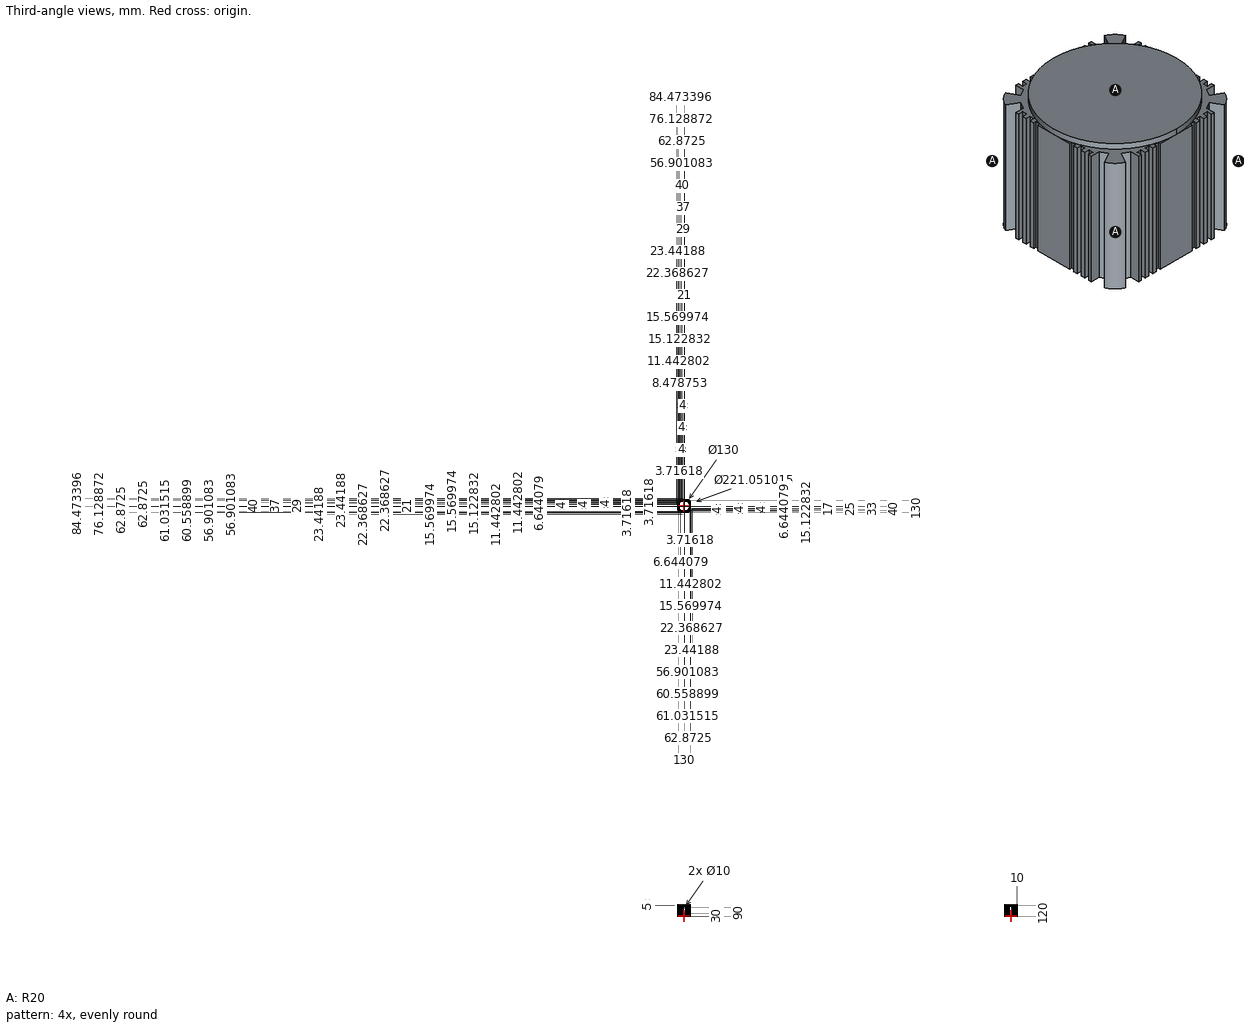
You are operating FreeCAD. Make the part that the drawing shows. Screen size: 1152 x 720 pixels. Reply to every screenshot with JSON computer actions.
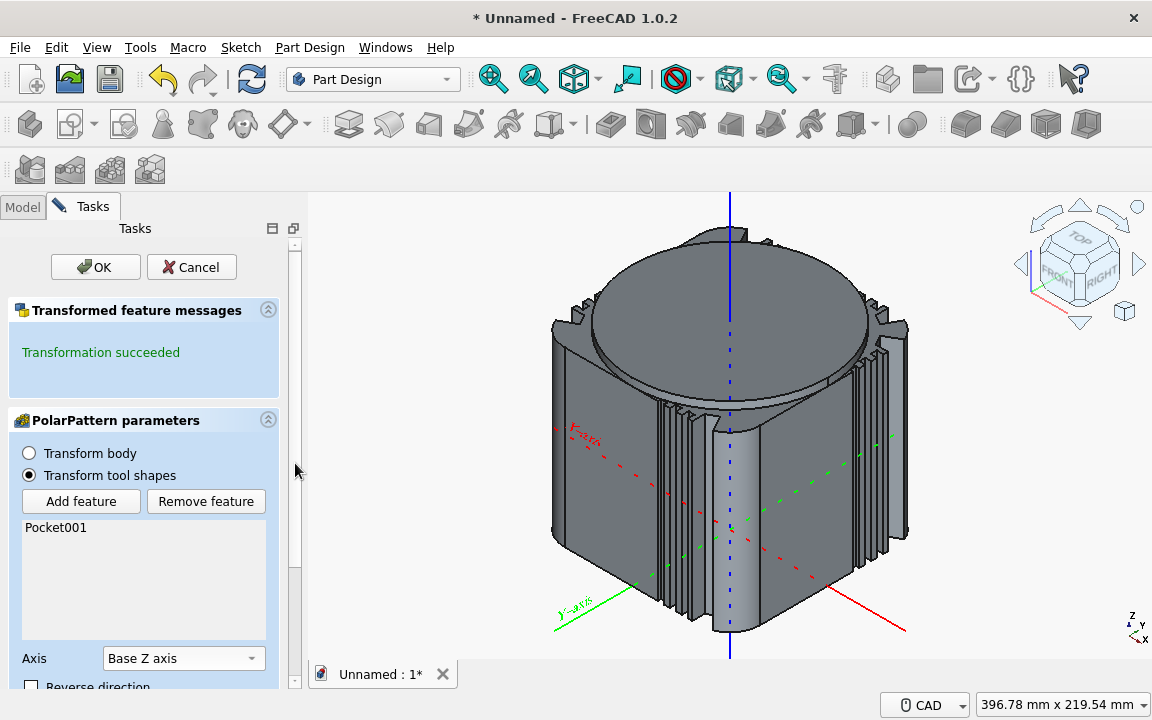
{"action": "left_click", "coordinate": [96, 267]}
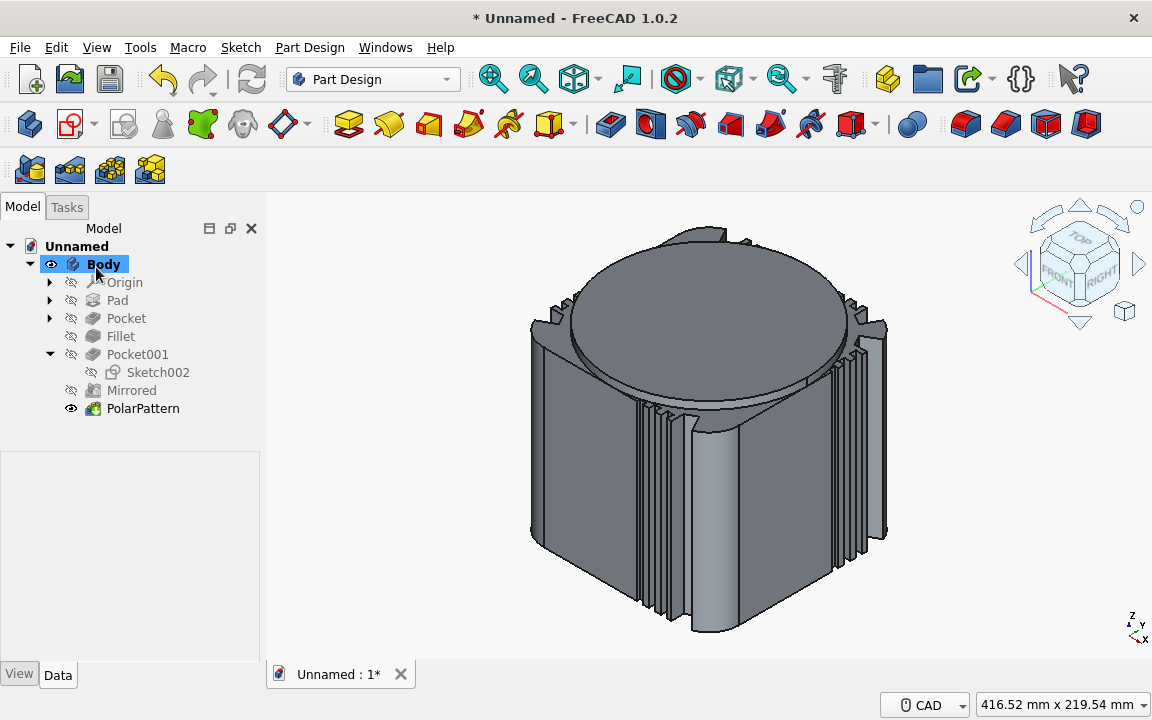
{"action": "left_click", "coordinate": [709, 418]}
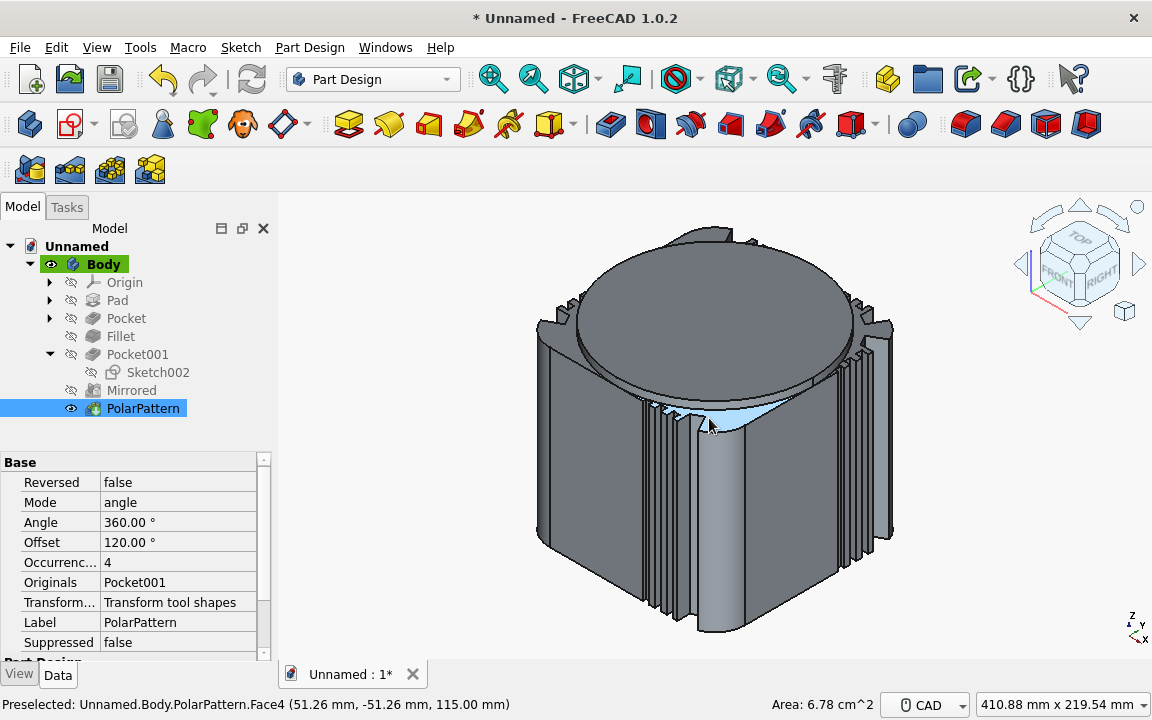
{"action": "left_click", "coordinate": [70, 124]}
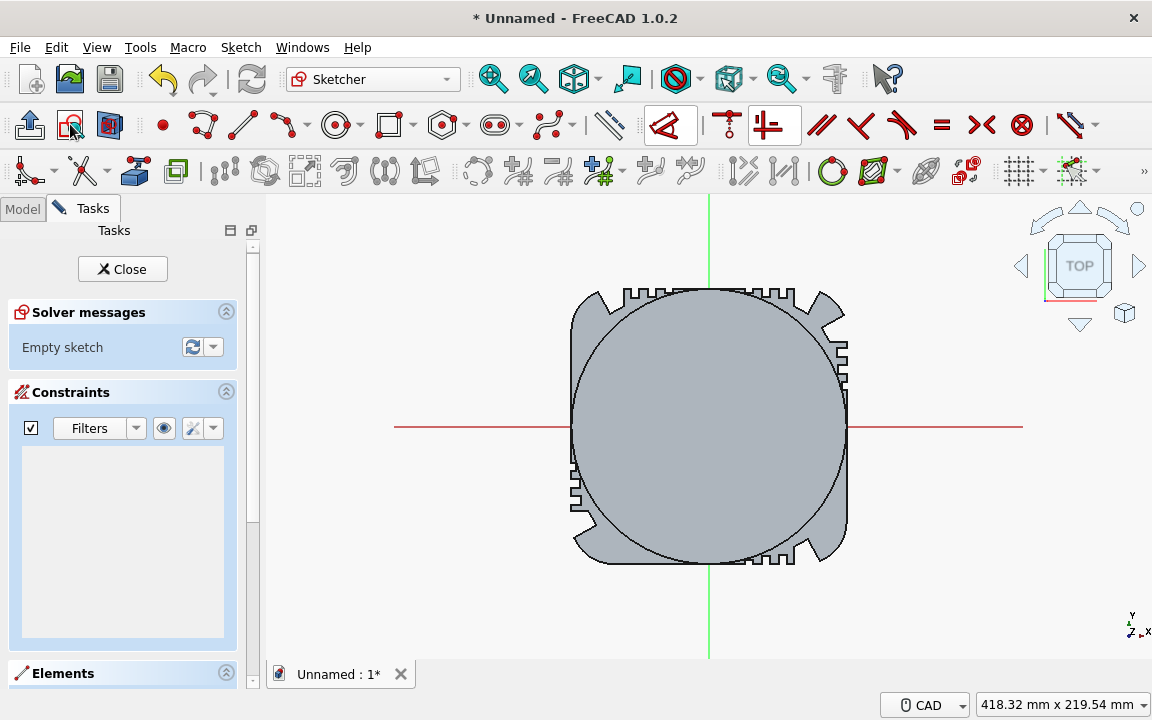
{"action": "scroll", "coordinate": [606, 334], "scroll_direction": "up", "scroll_amount": 5}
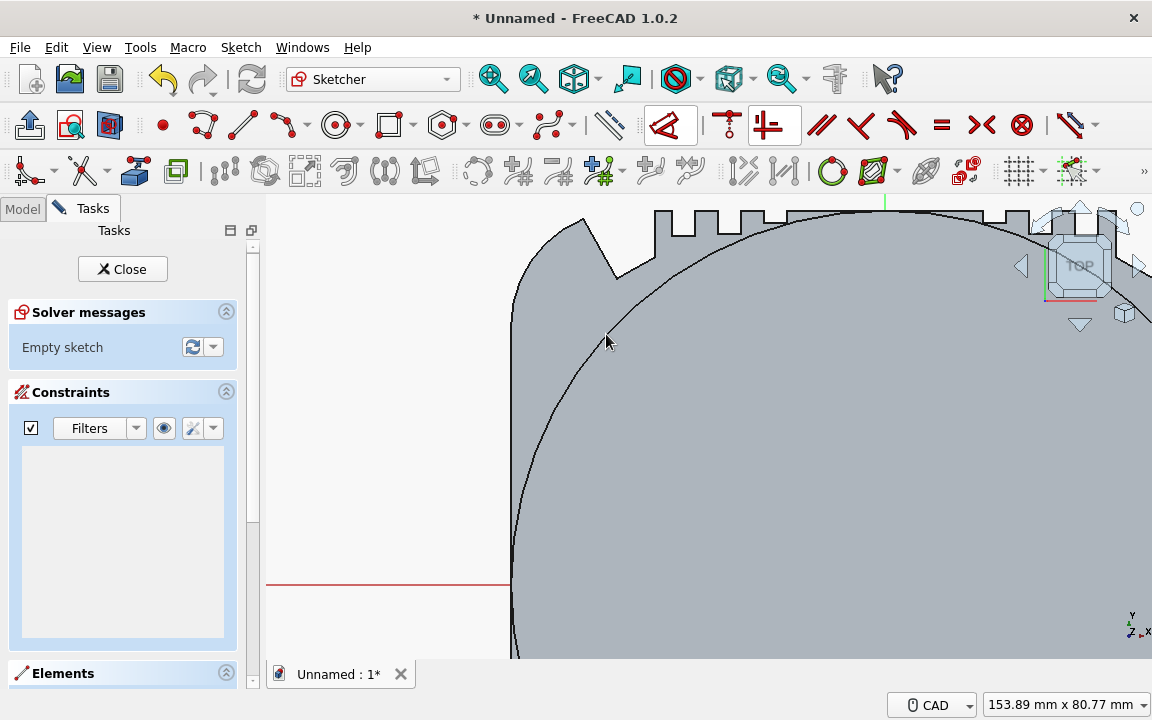
{"action": "left_click", "coordinate": [204, 126]}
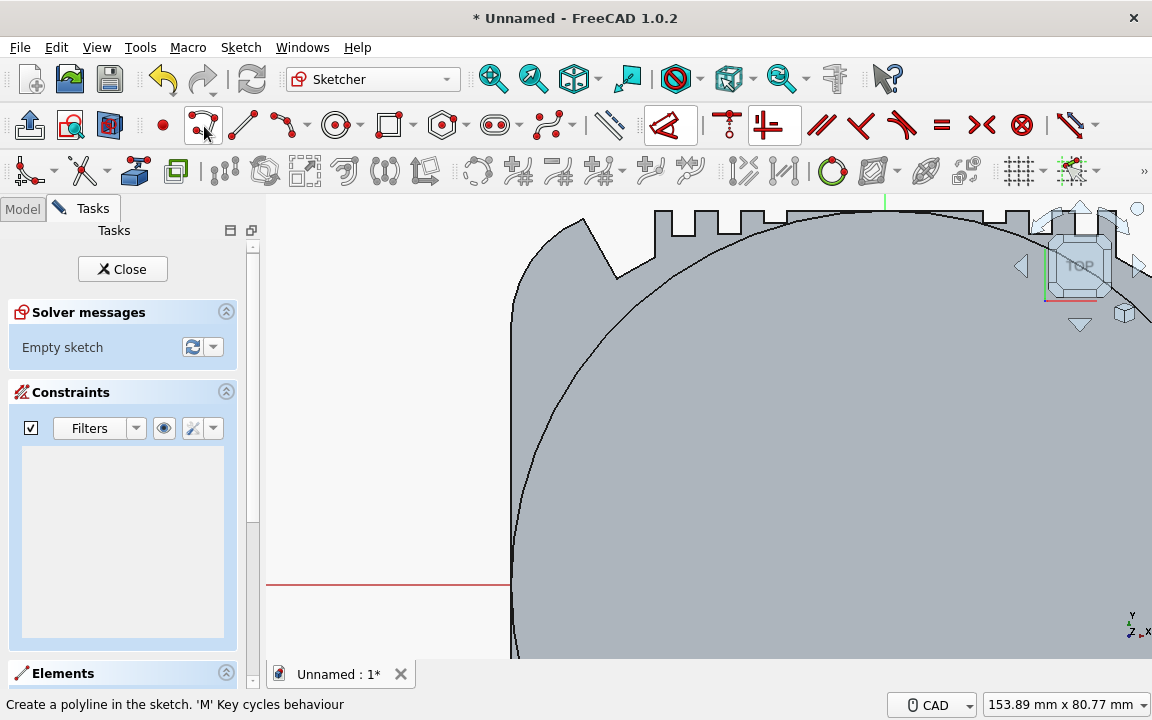
{"action": "left_click", "coordinate": [558, 355]}
{"action": "left_click", "coordinate": [579, 316]}
{"action": "left_click", "coordinate": [492, 268]}
{"action": "left_click", "coordinate": [492, 355]}
{"action": "left_click", "coordinate": [558, 356]}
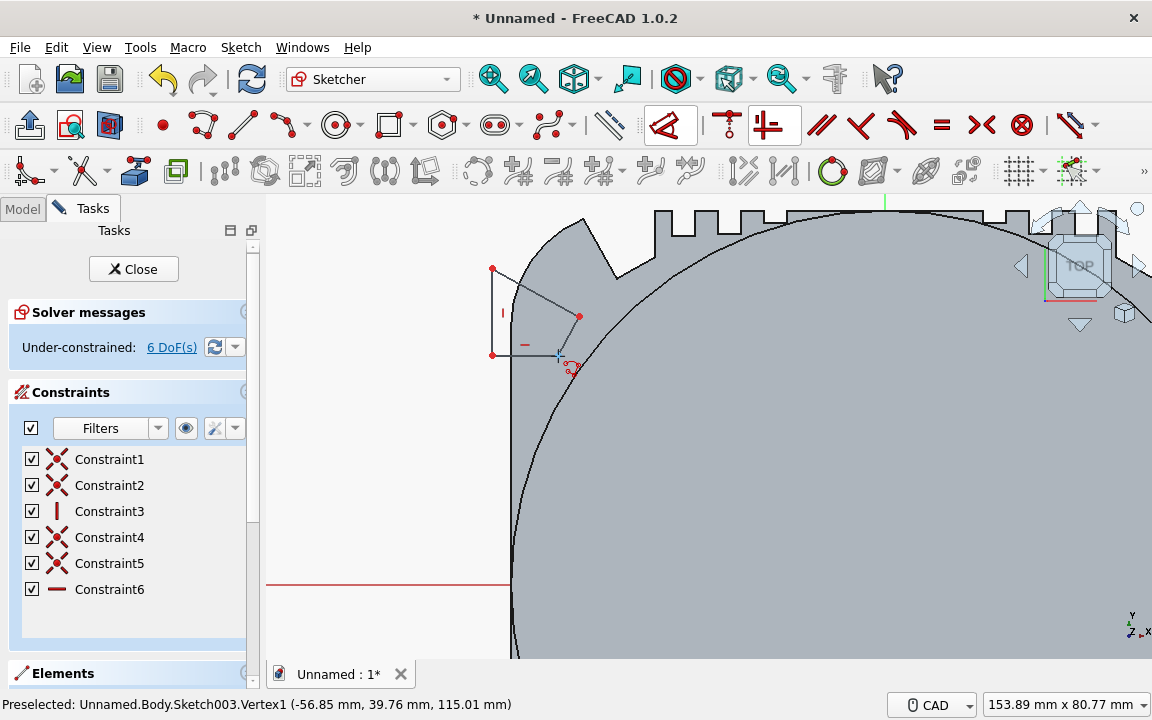
{"action": "left_click", "coordinate": [390, 126]}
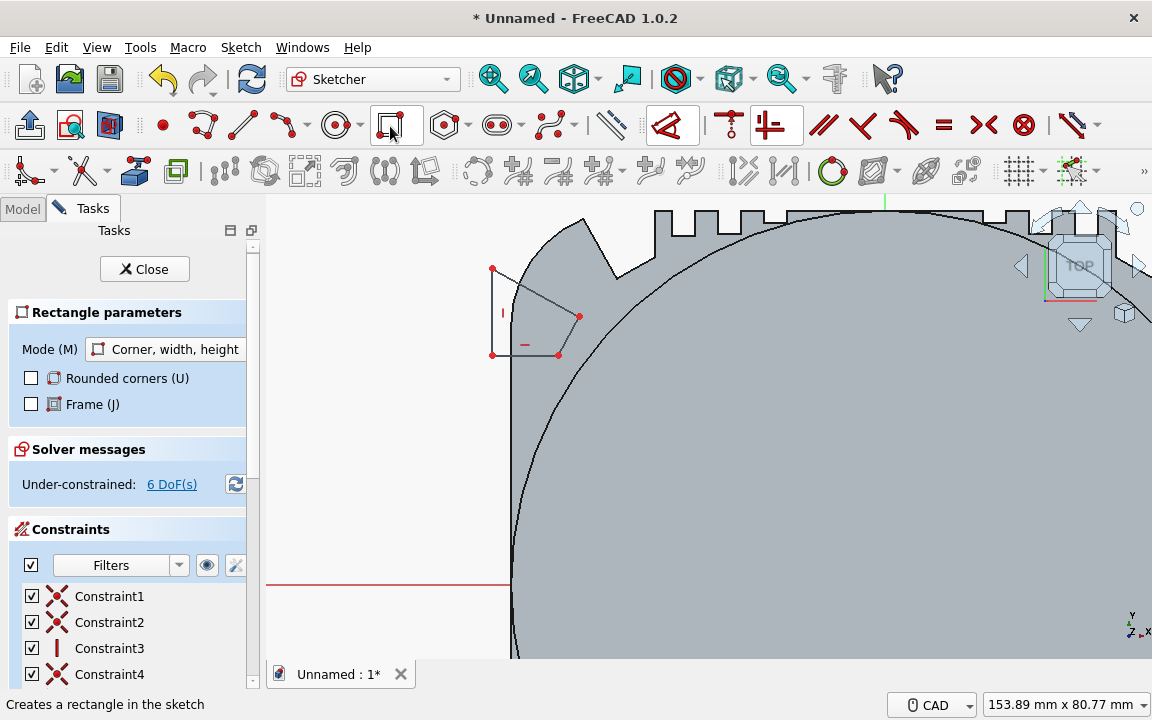
{"action": "left_click", "coordinate": [447, 372]}
{"action": "mouse_move", "coordinate": [537, 395]}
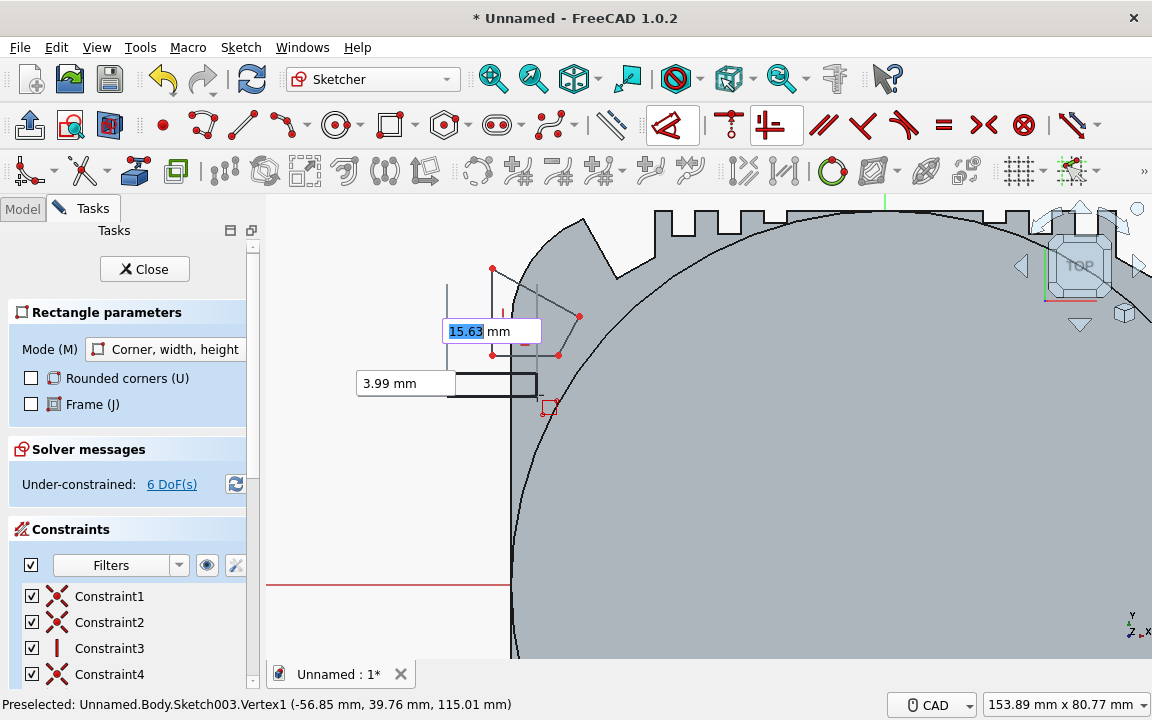
{"action": "type", "text": "15.569974"}
{"action": "key", "text": "Tab"}
{"action": "type", "text": "4"}
{"action": "key", "text": "Return"}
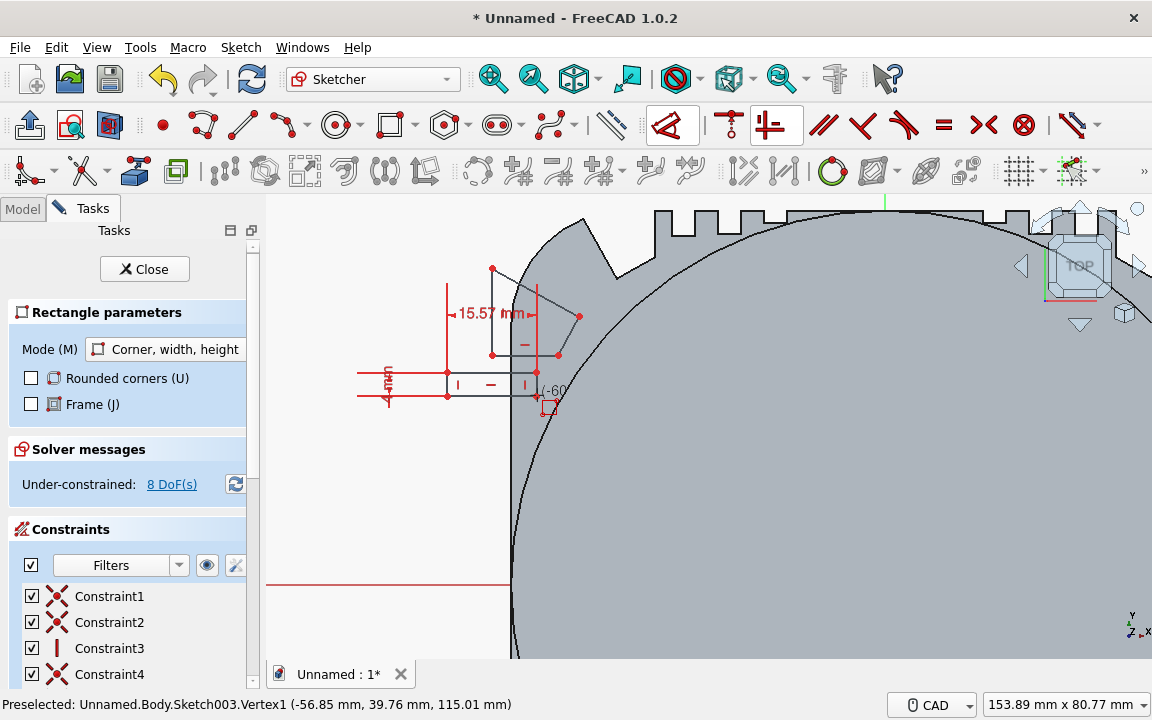
{"action": "left_click", "coordinate": [399, 418]}
{"action": "mouse_move", "coordinate": [534, 441]}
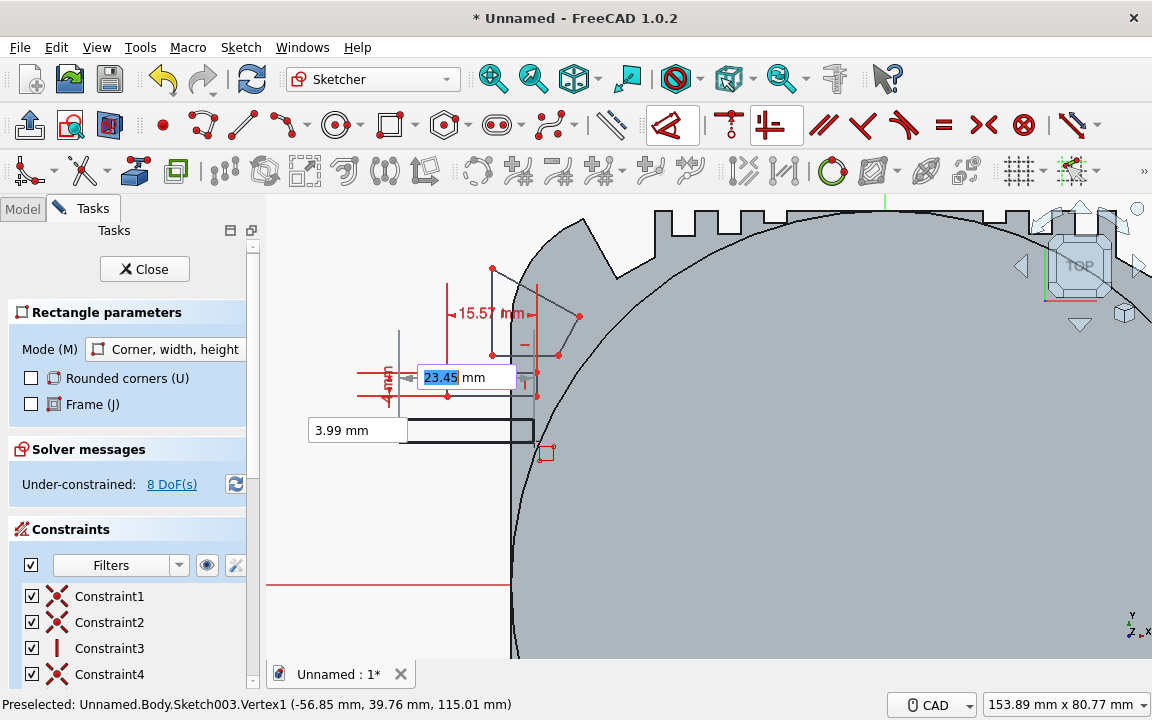
{"action": "type", "text": "23.44188"}
{"action": "key", "text": "Tab"}
{"action": "type", "text": "4"}
{"action": "key", "text": "Return"}